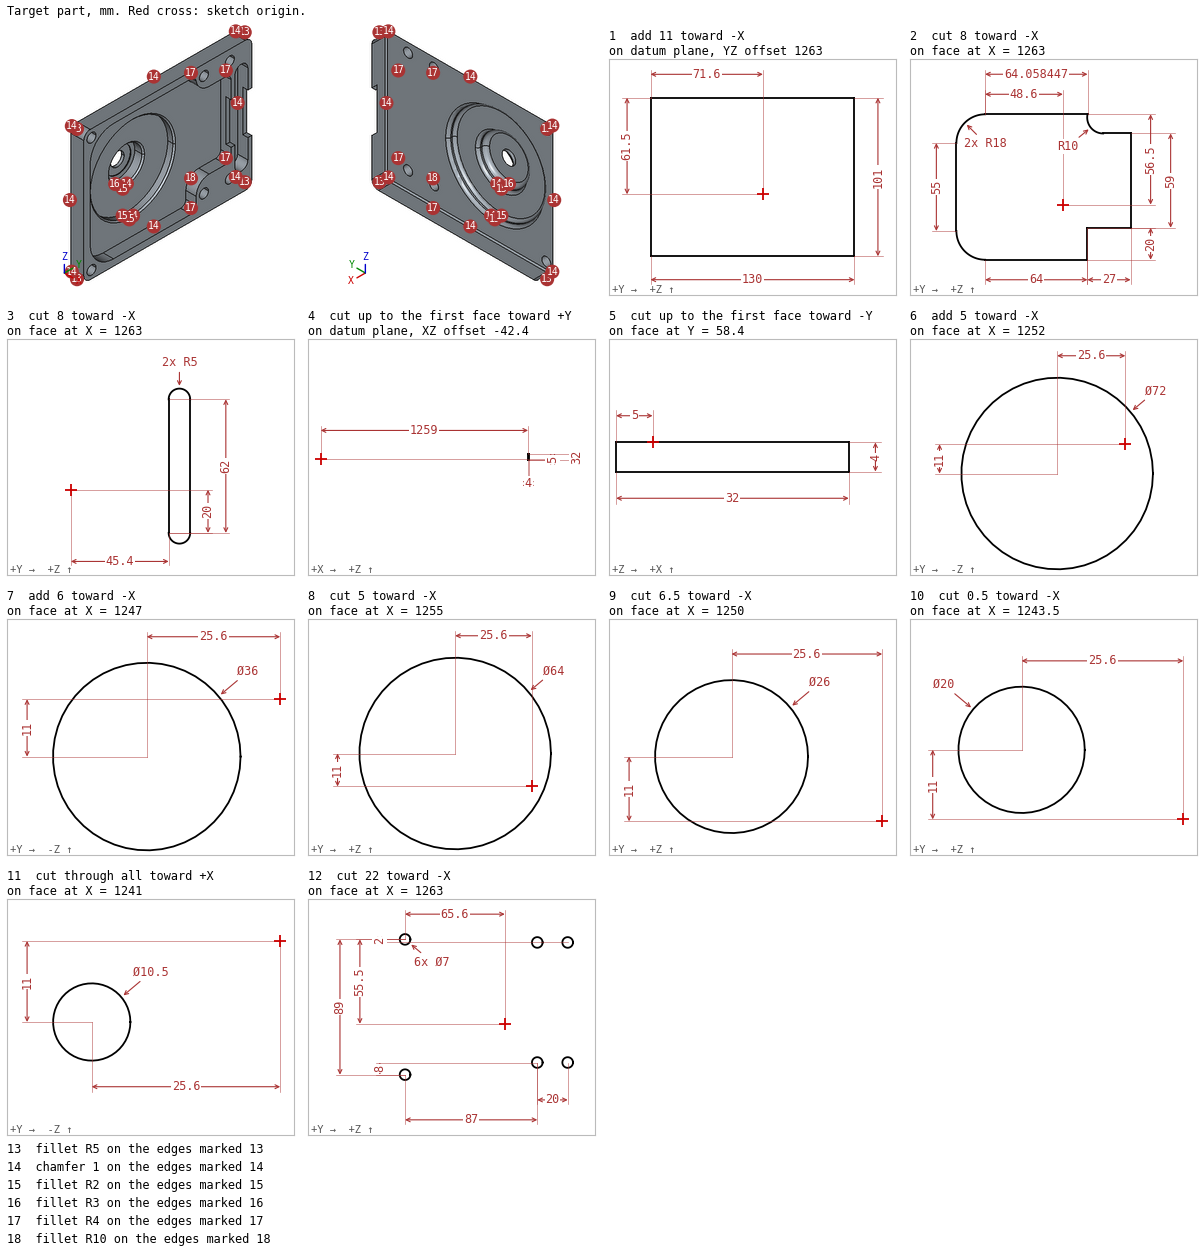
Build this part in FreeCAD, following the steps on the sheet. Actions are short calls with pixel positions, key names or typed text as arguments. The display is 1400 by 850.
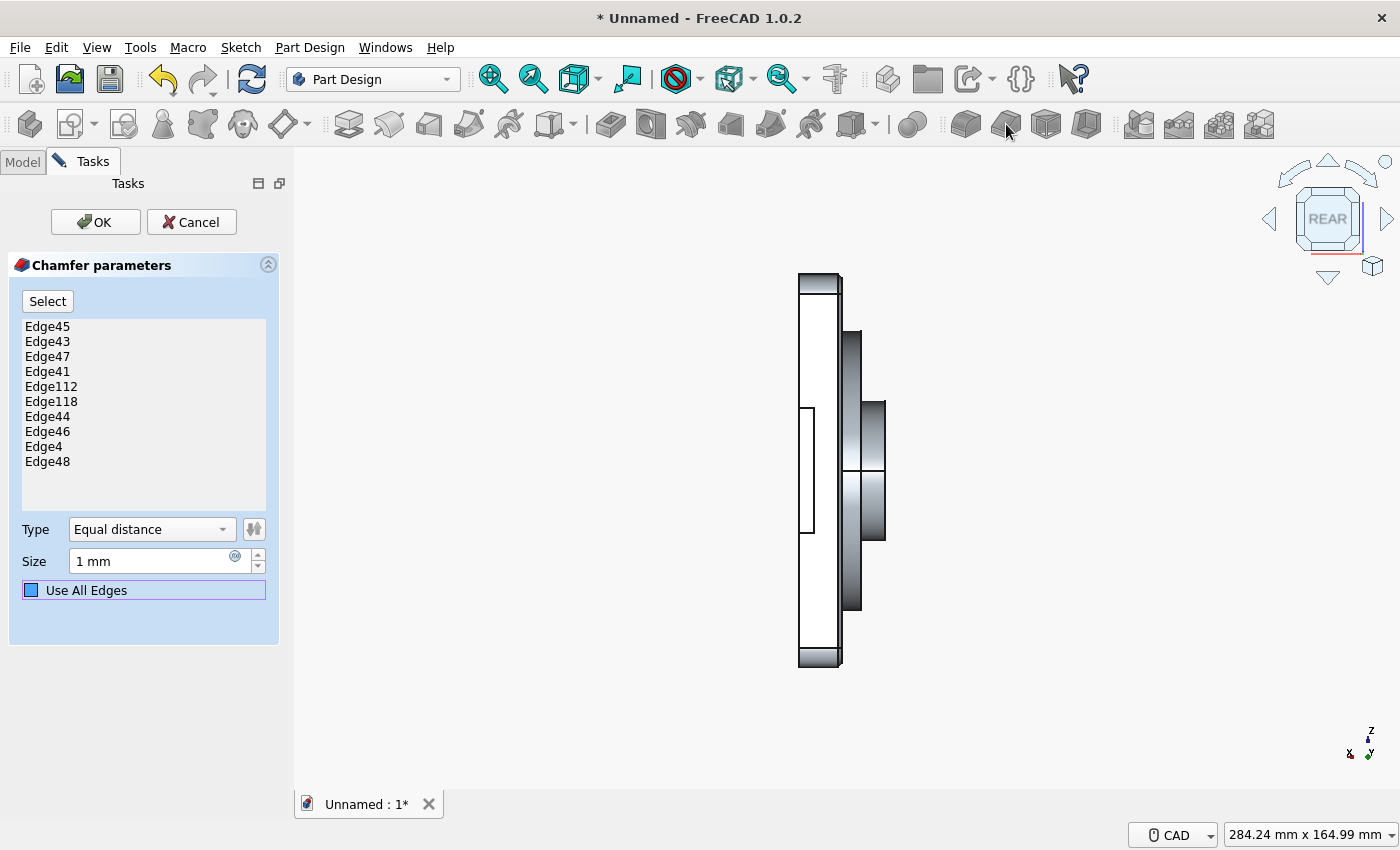
click(96, 222)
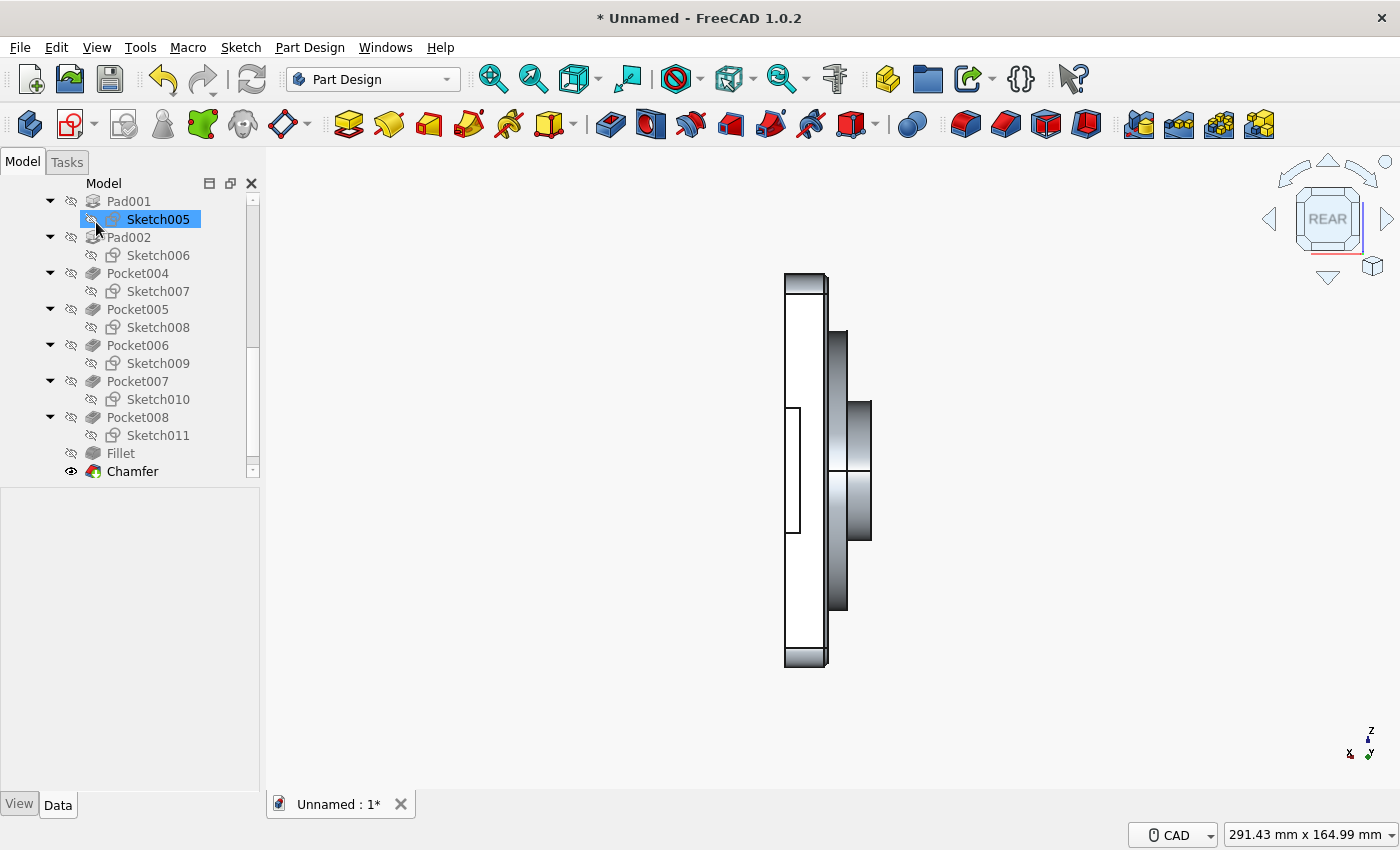
click(847, 552)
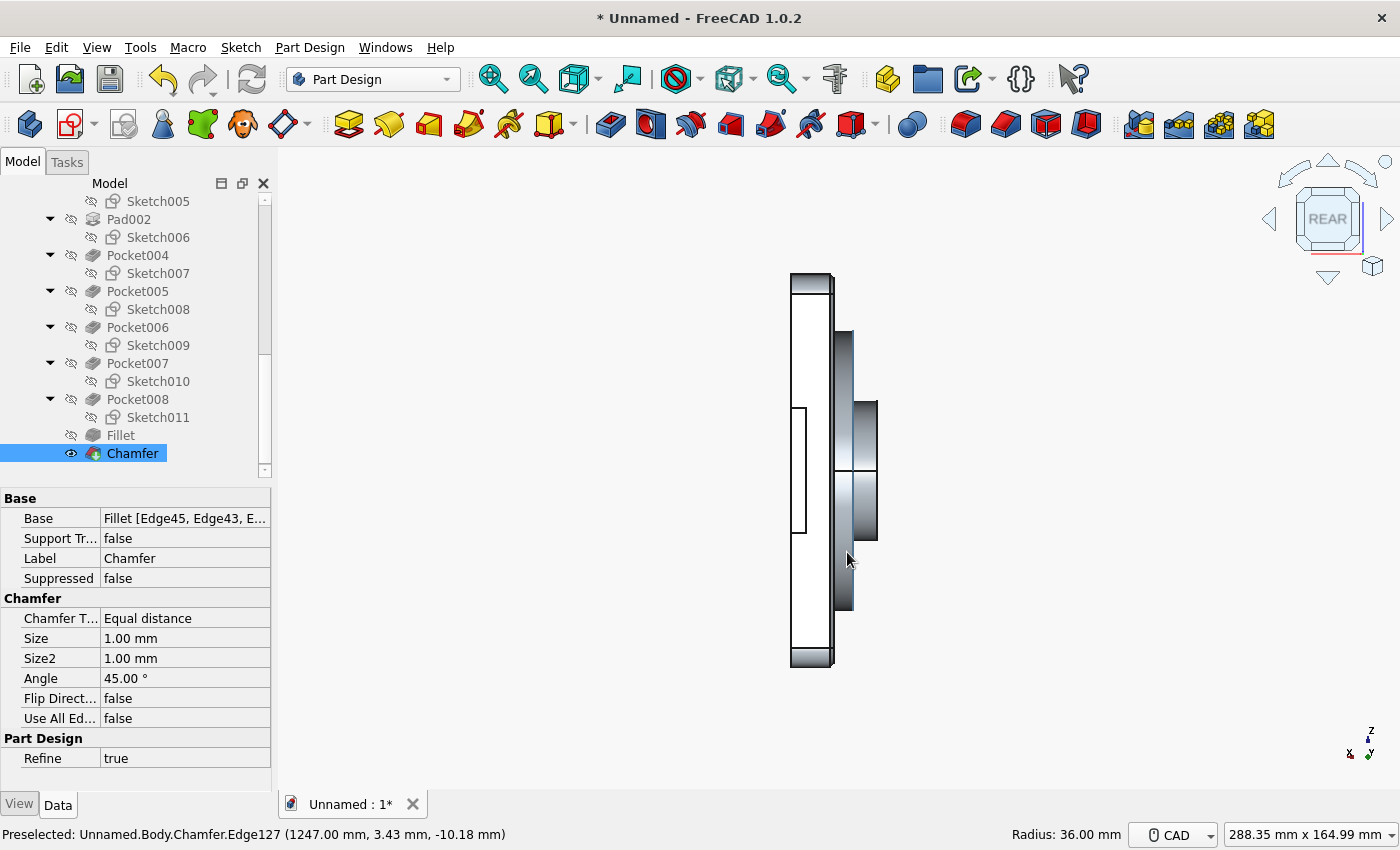
key(0)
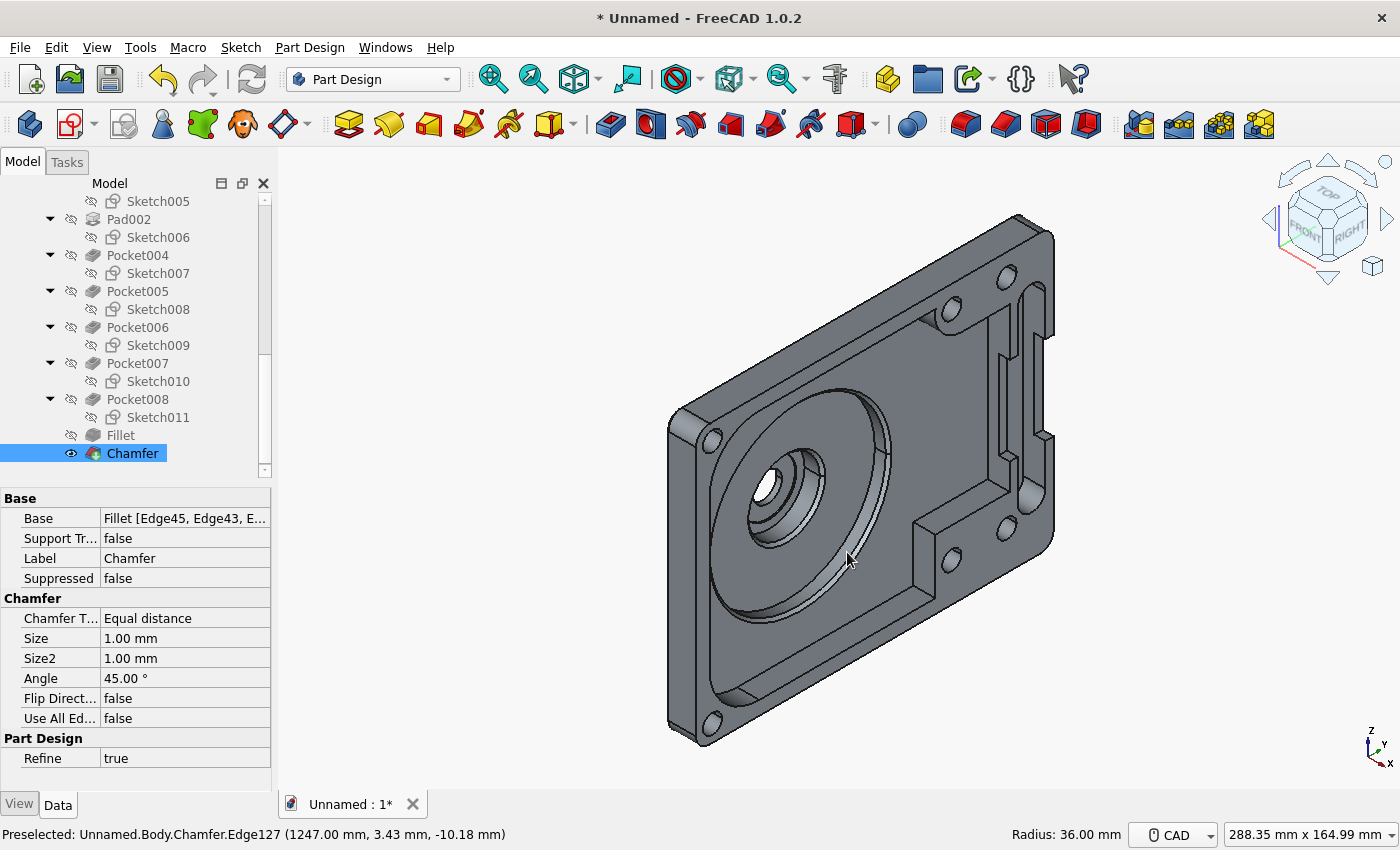
key(2)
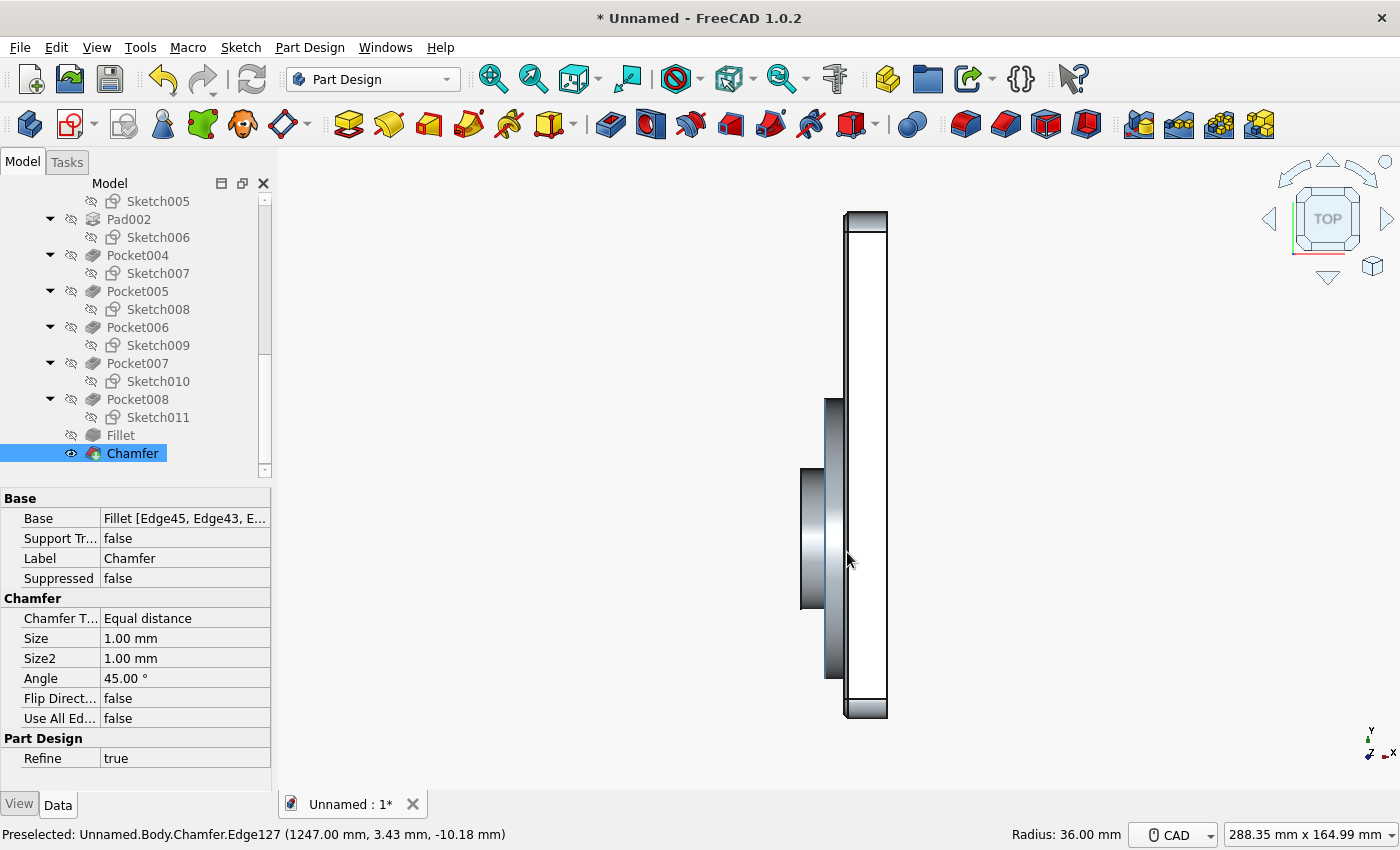
key(1)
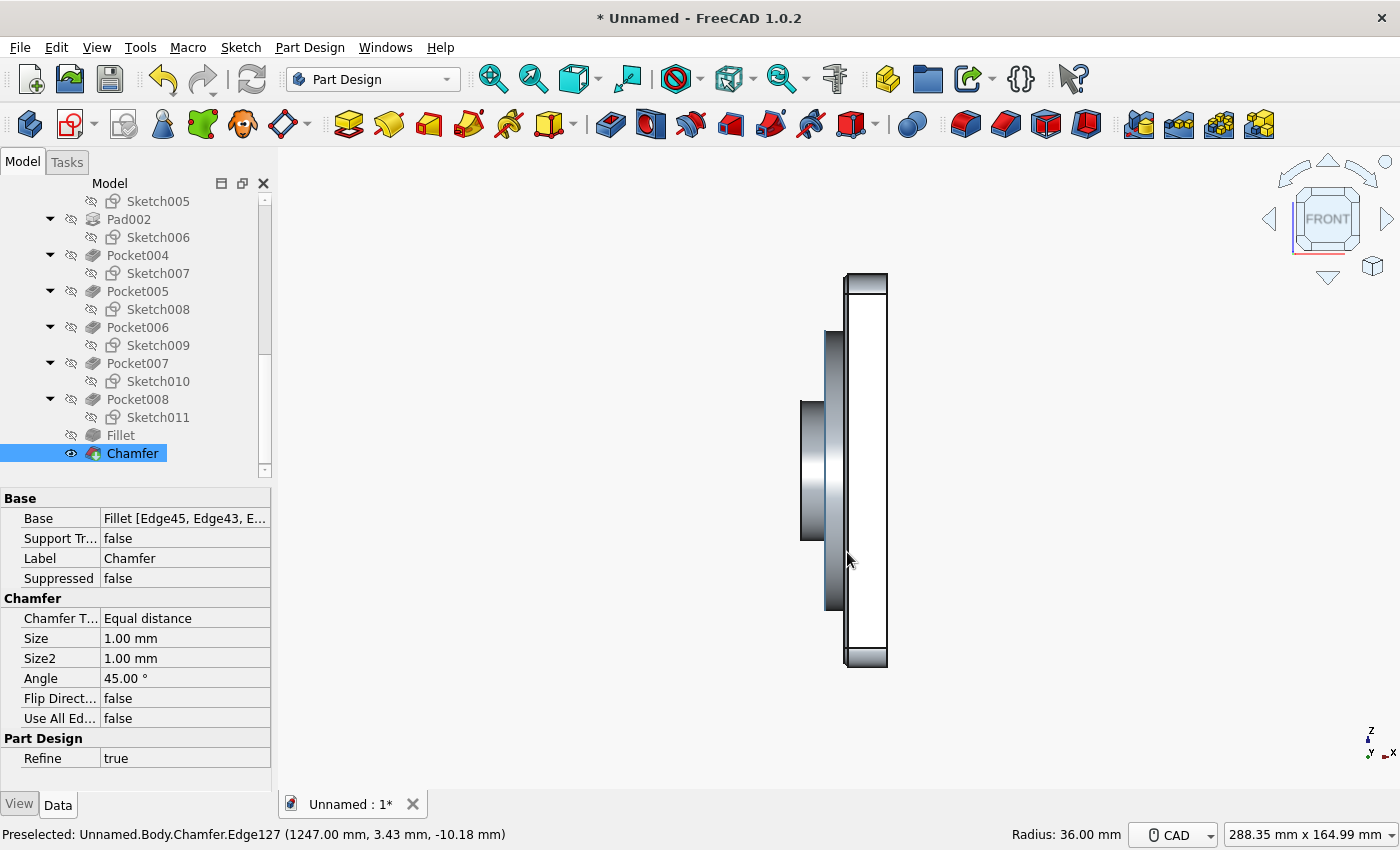
key(3)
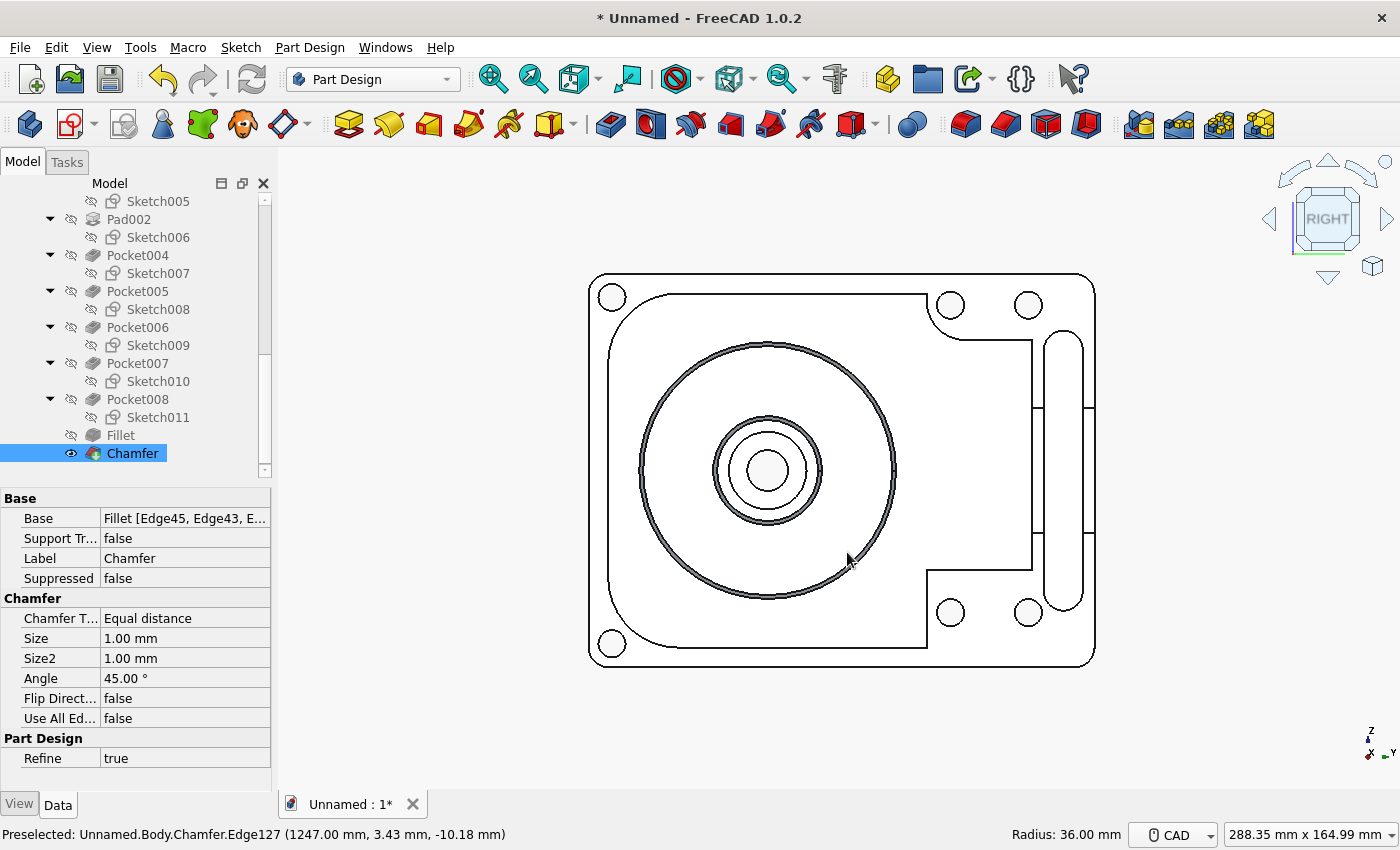
key(5)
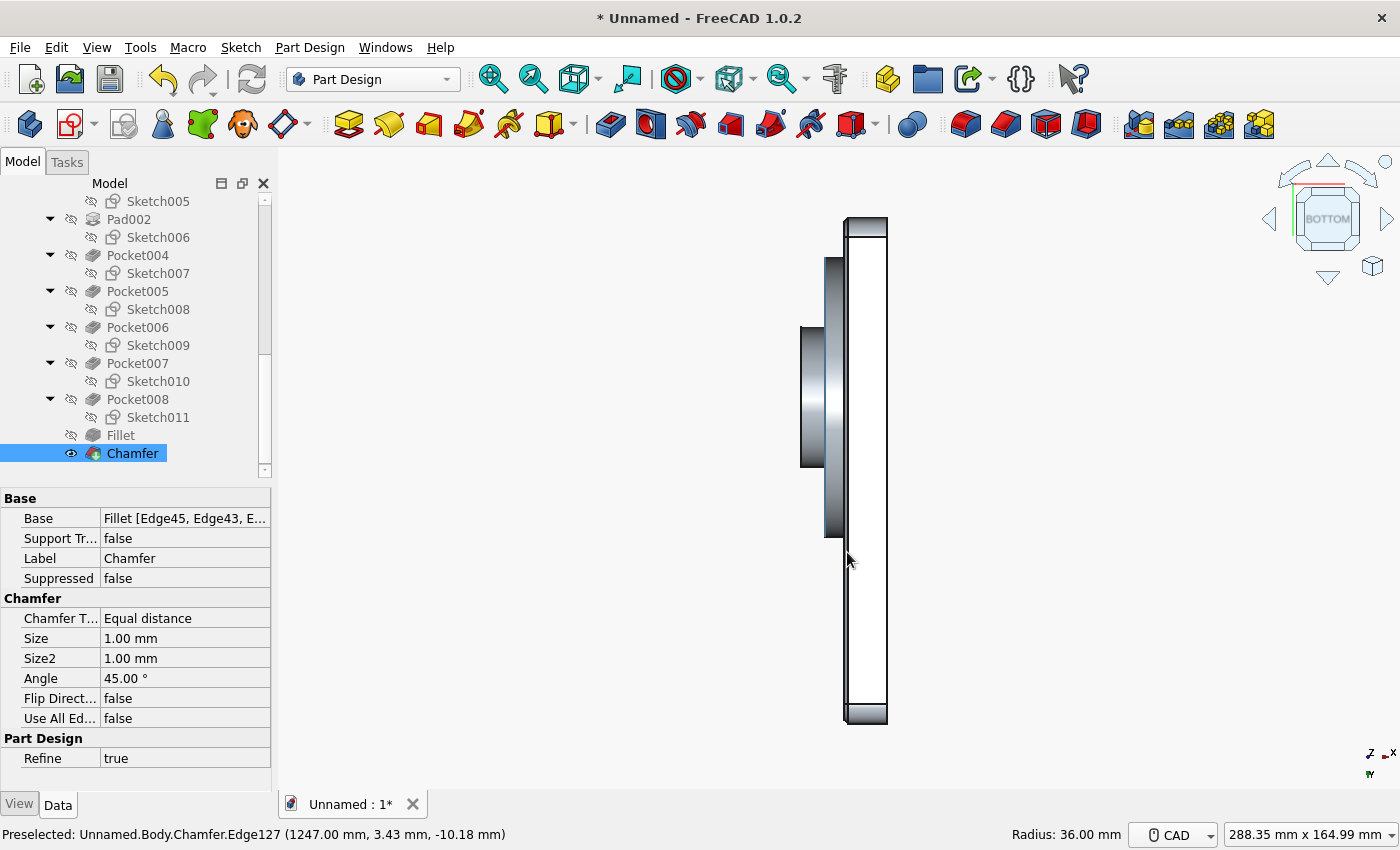
key(4)